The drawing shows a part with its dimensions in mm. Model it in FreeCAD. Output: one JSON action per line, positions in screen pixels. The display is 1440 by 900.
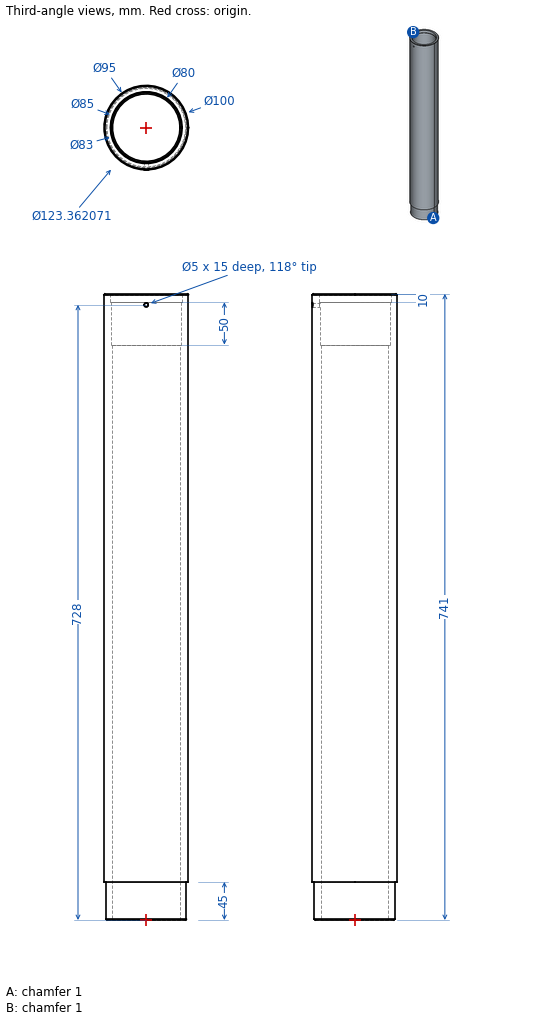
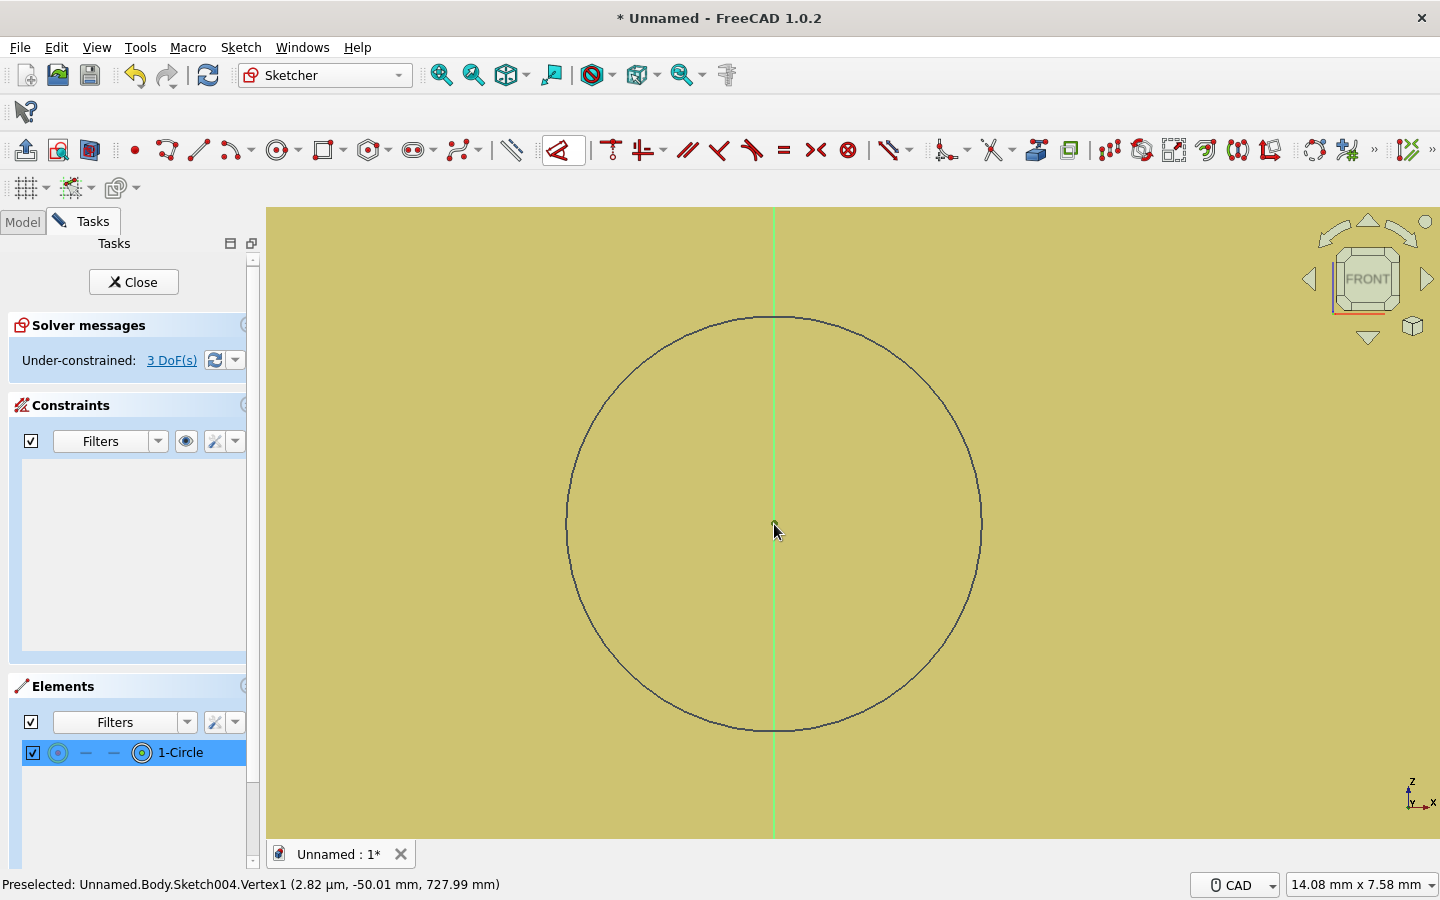
{"action": "left_click", "coordinate": [774, 770]}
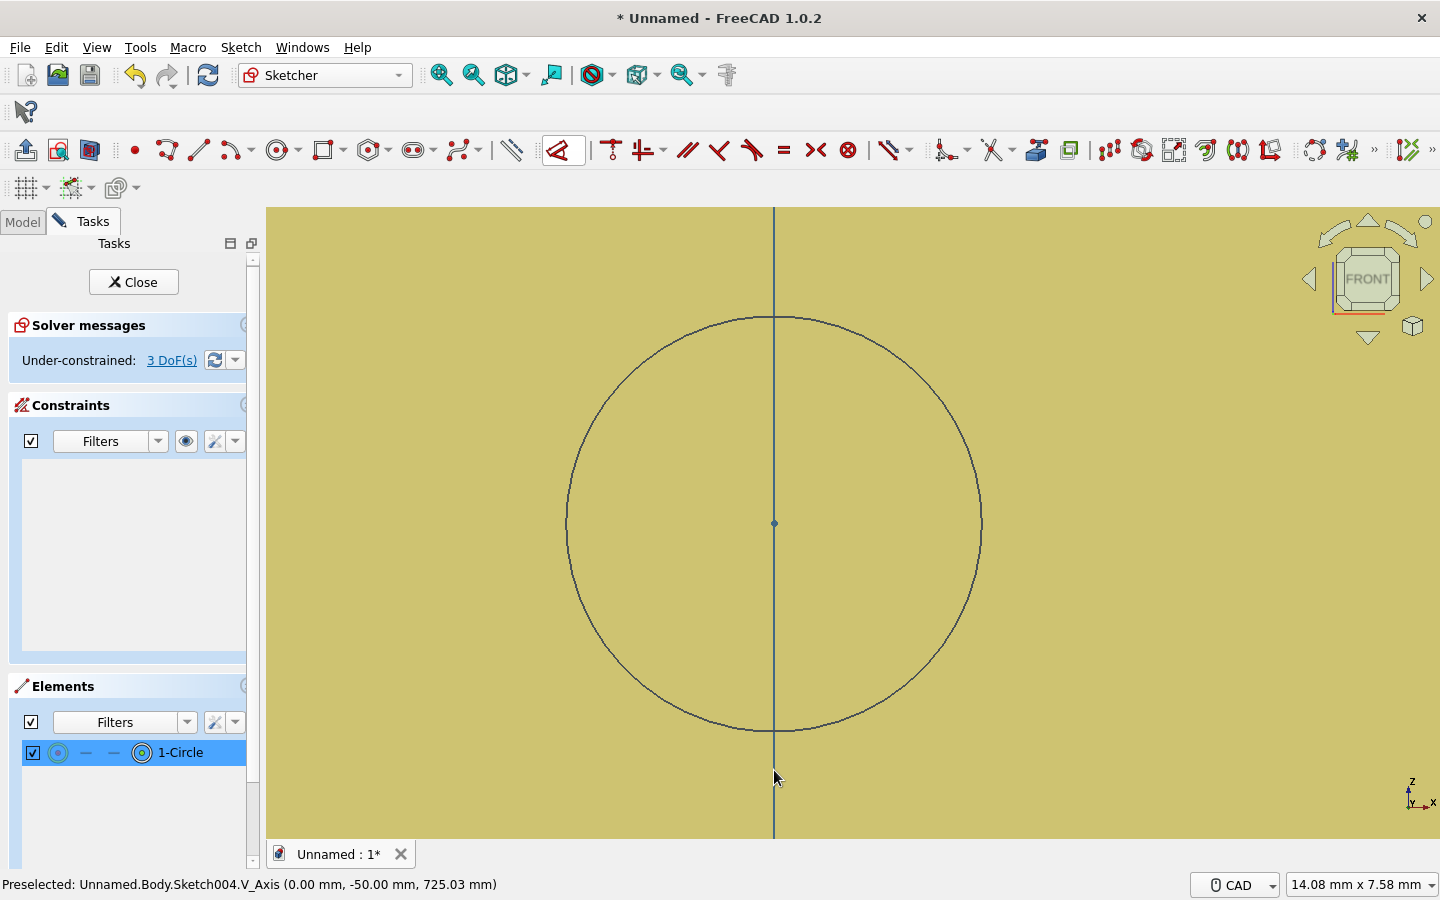
{"action": "left_click", "coordinate": [612, 150]}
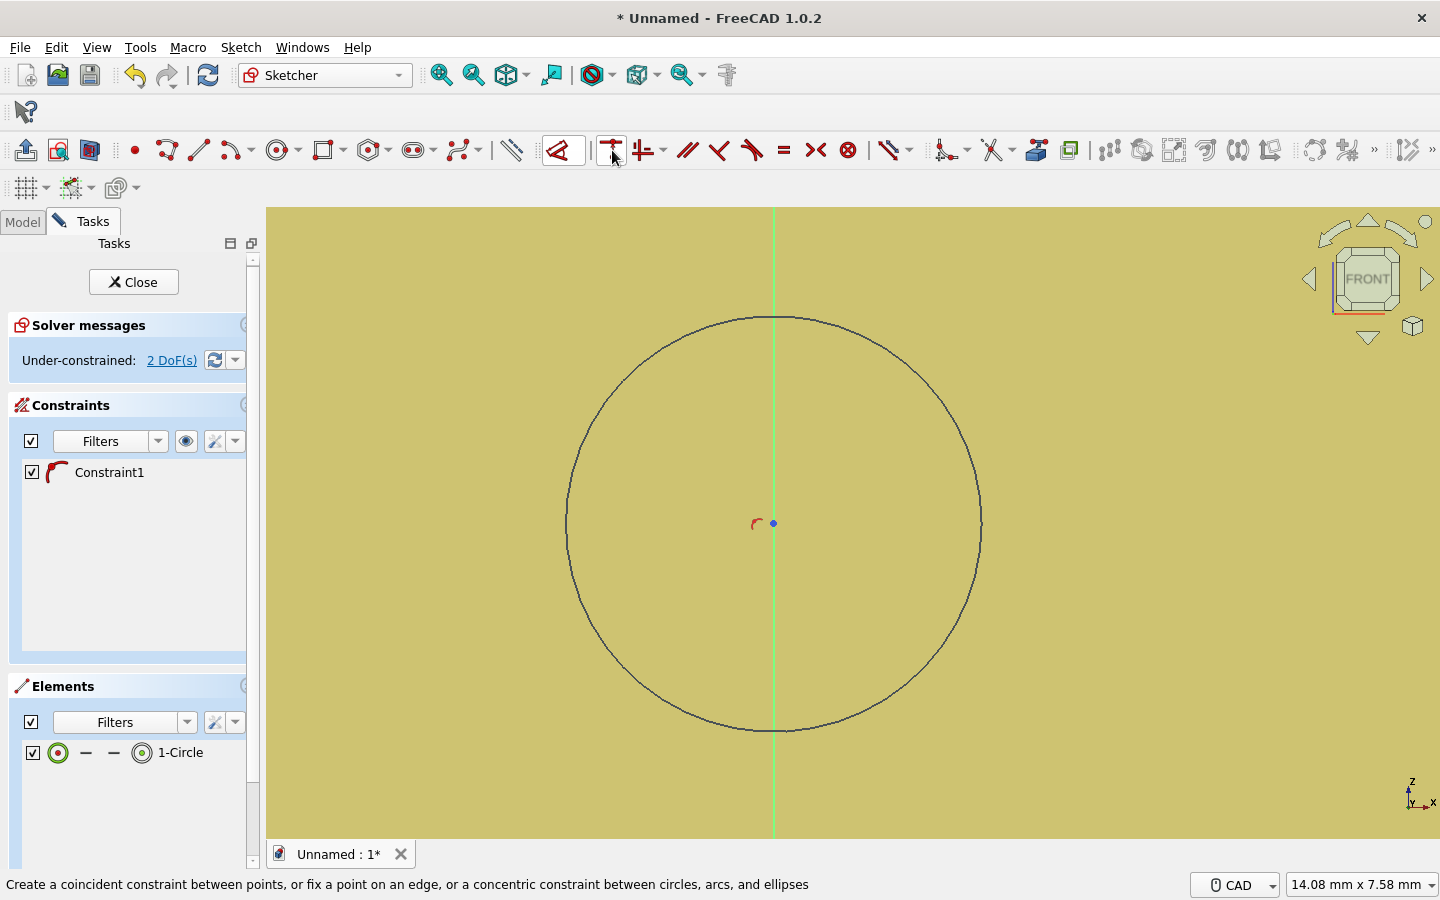
{"action": "left_click", "coordinate": [920, 377]}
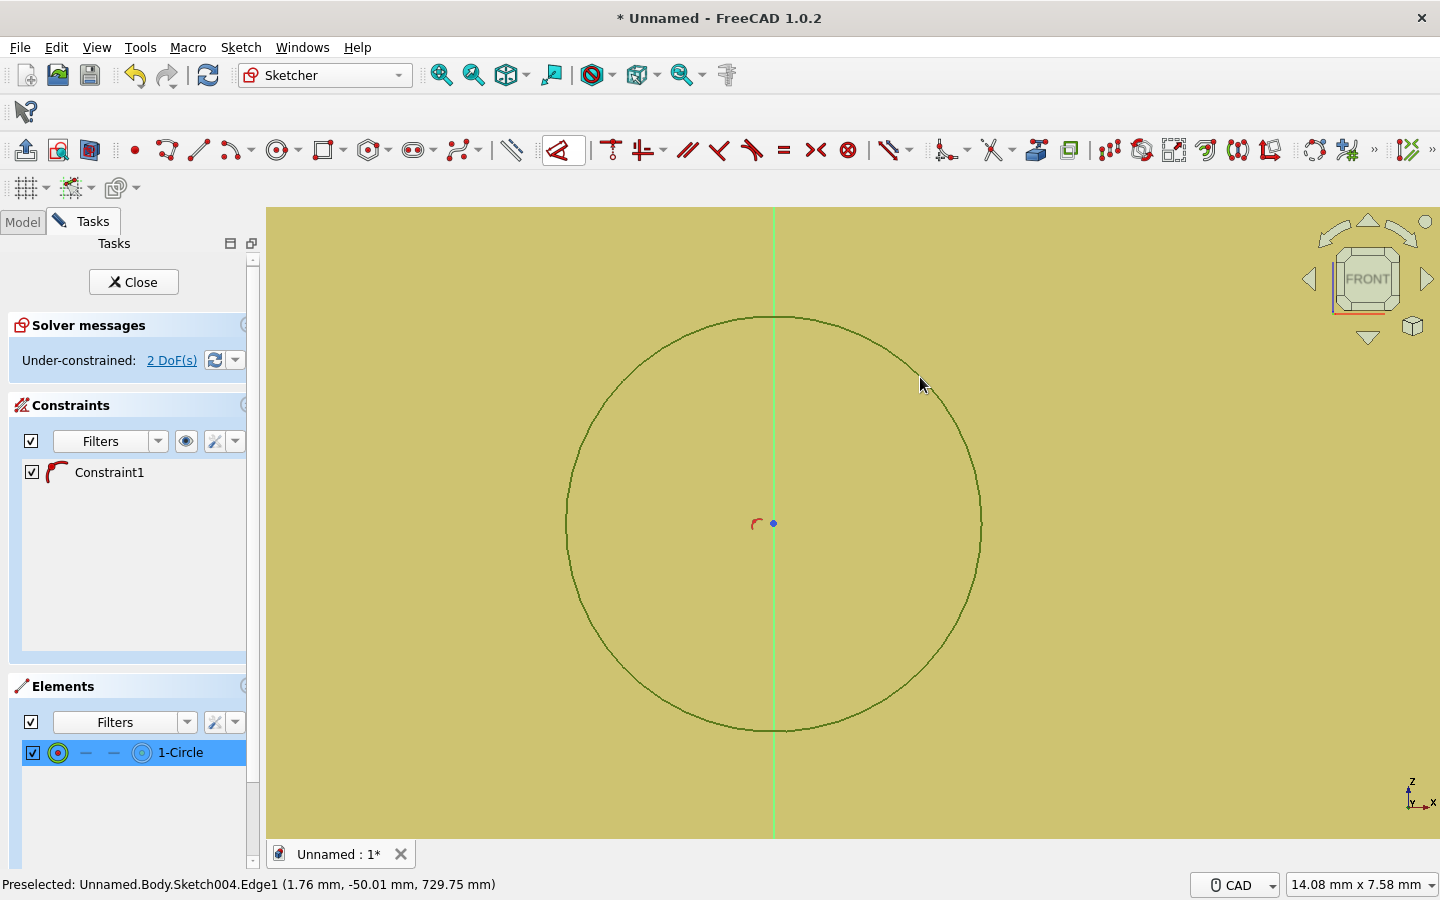
{"action": "key", "text": "k o"}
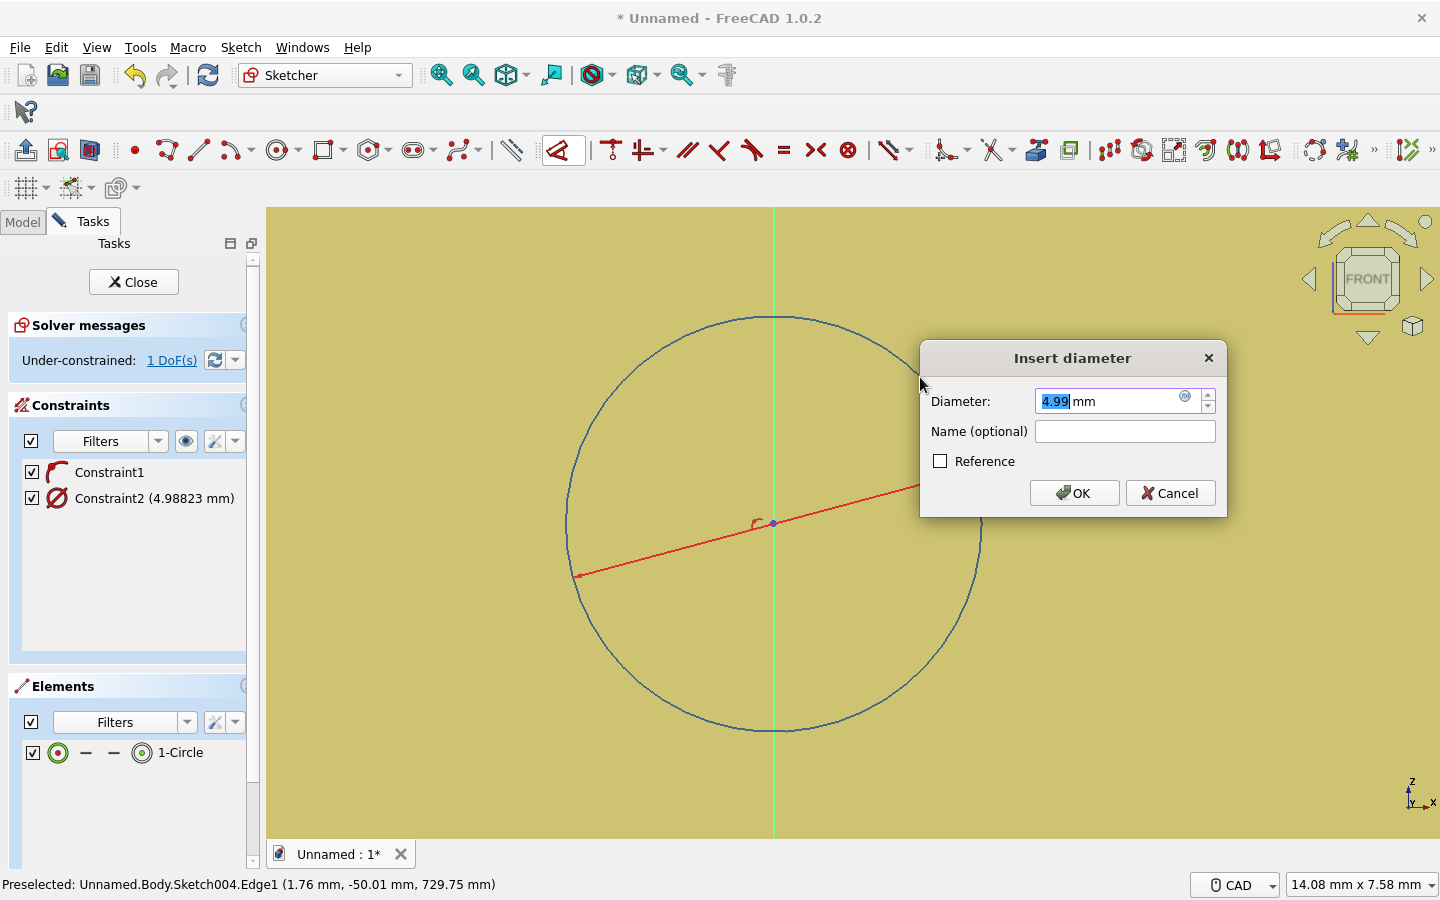
{"action": "type", "text": "5"}
{"action": "key", "text": "Return"}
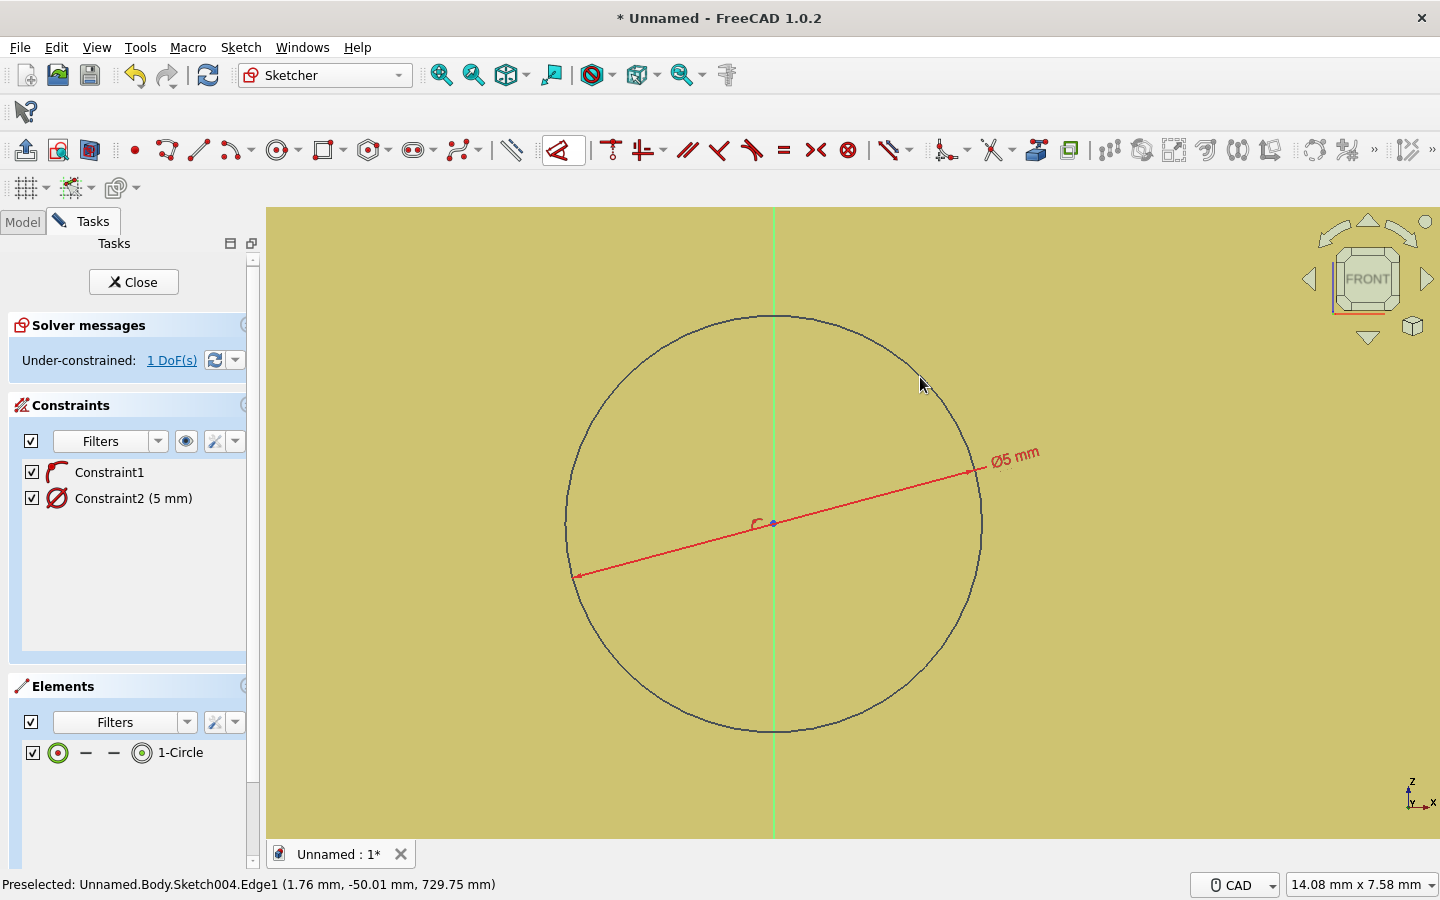
{"action": "left_click", "coordinate": [774, 524]}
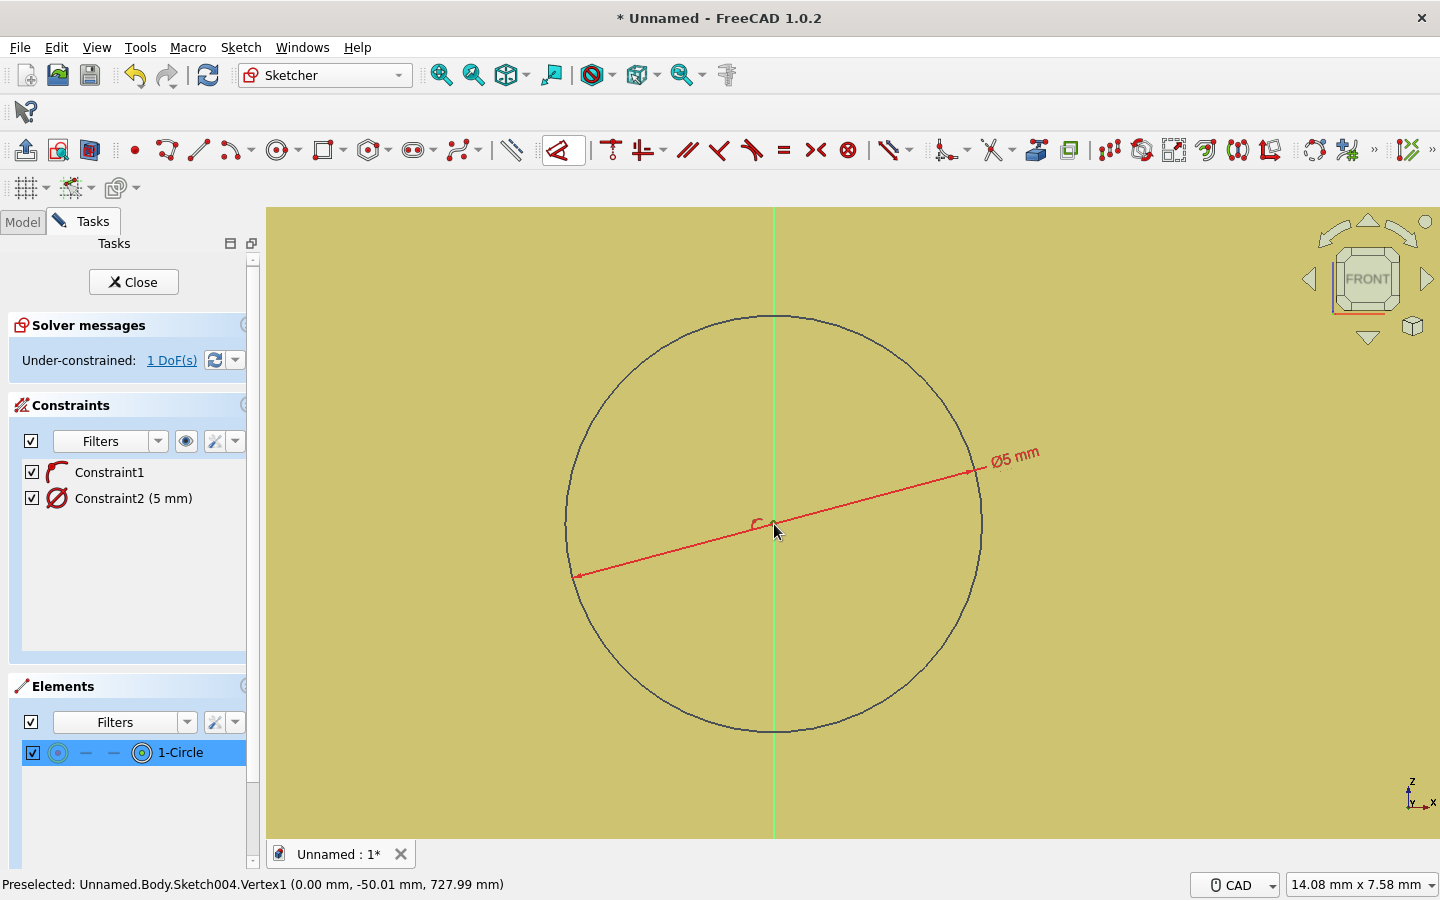
{"action": "key", "text": "i"}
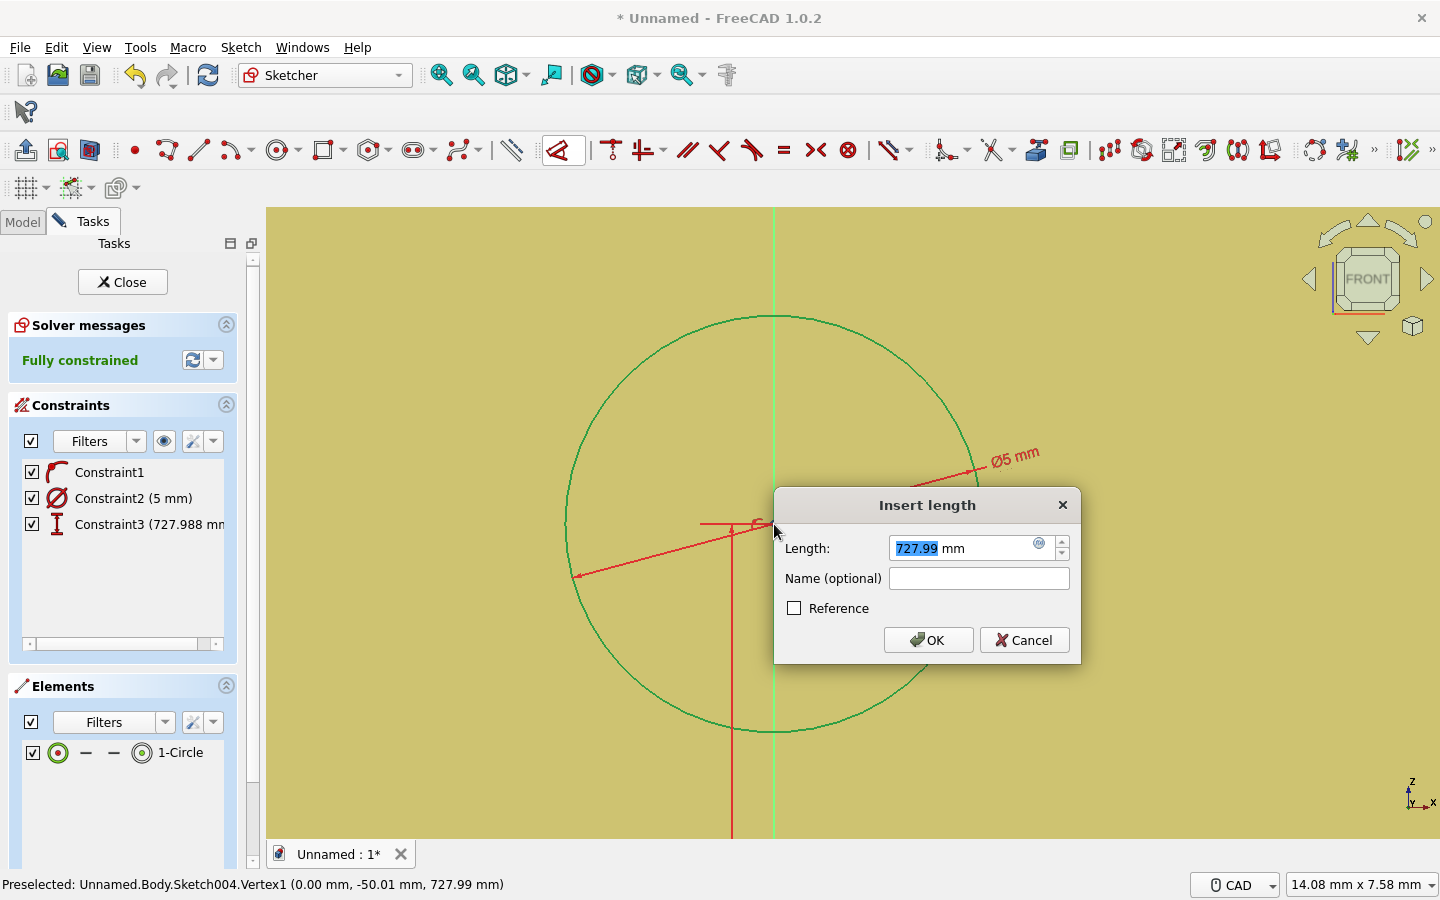
{"action": "type", "text": "728"}
{"action": "key", "text": "Return"}